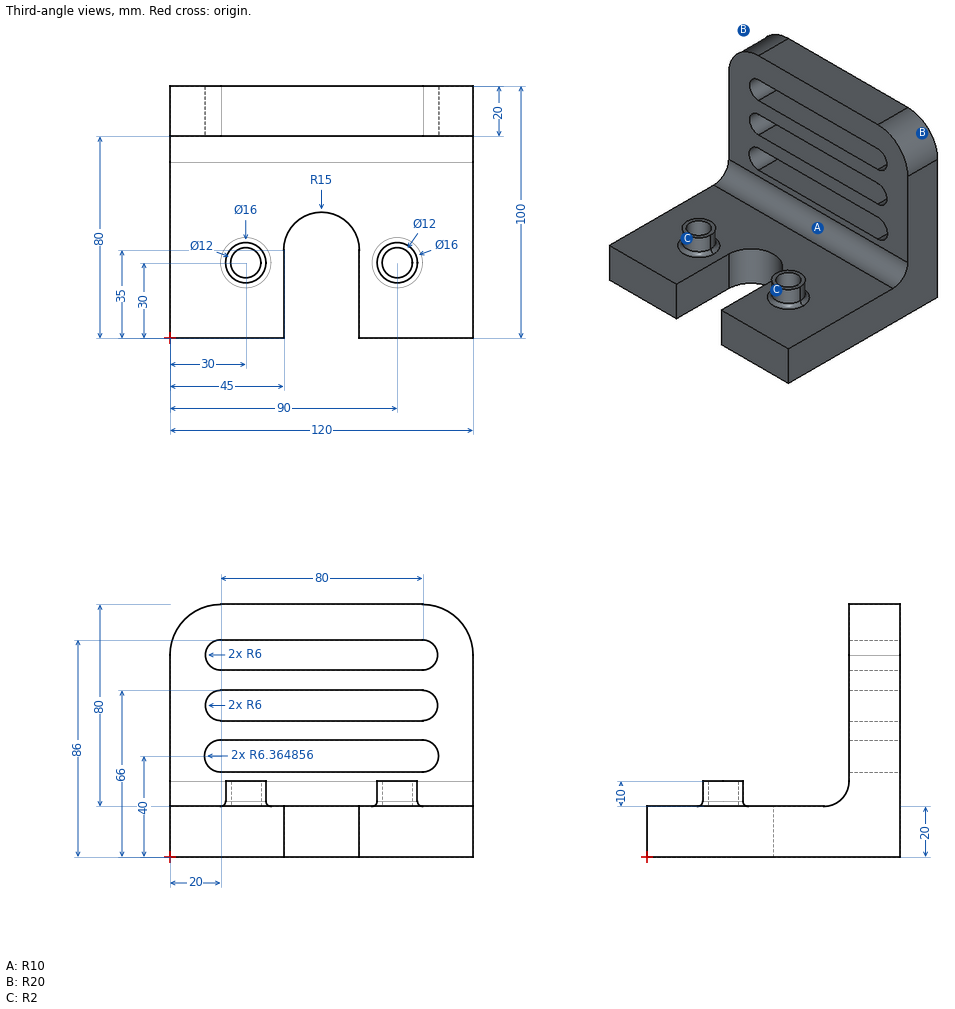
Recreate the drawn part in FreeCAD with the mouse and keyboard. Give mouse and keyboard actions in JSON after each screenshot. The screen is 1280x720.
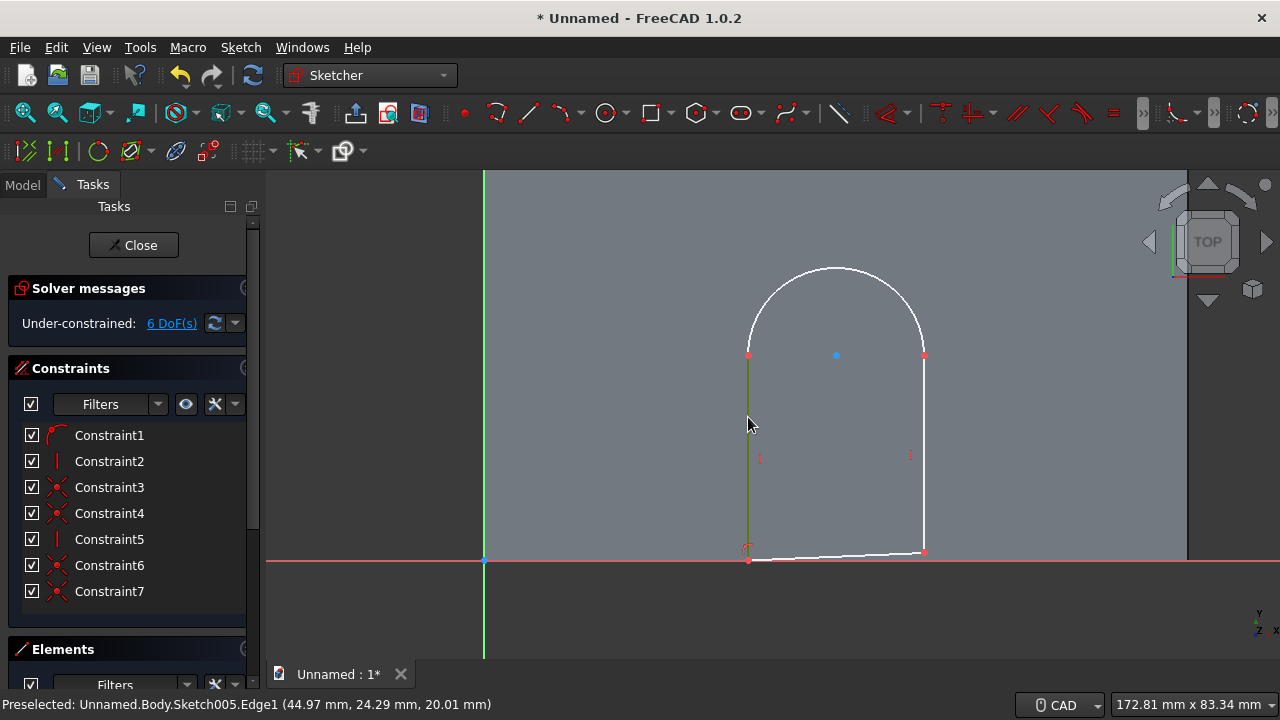
{"action": "left_click", "coordinate": [888, 285]}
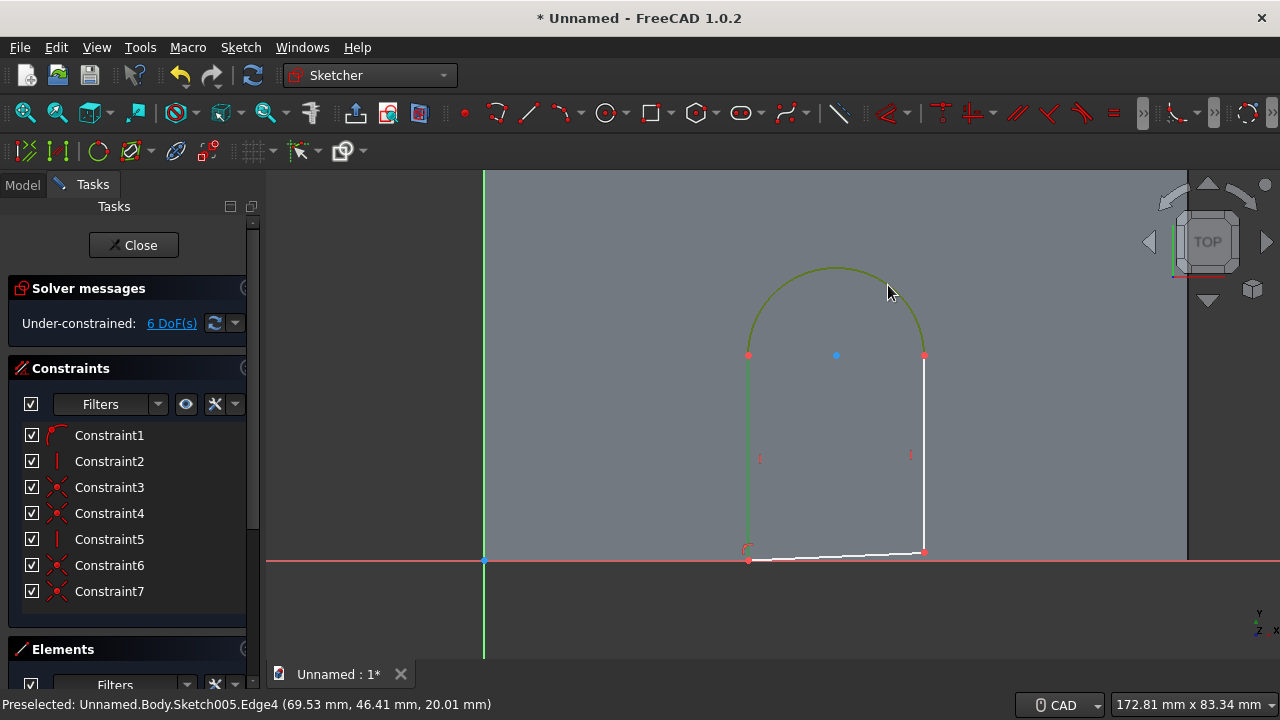
{"action": "left_click", "coordinate": [1082, 114]}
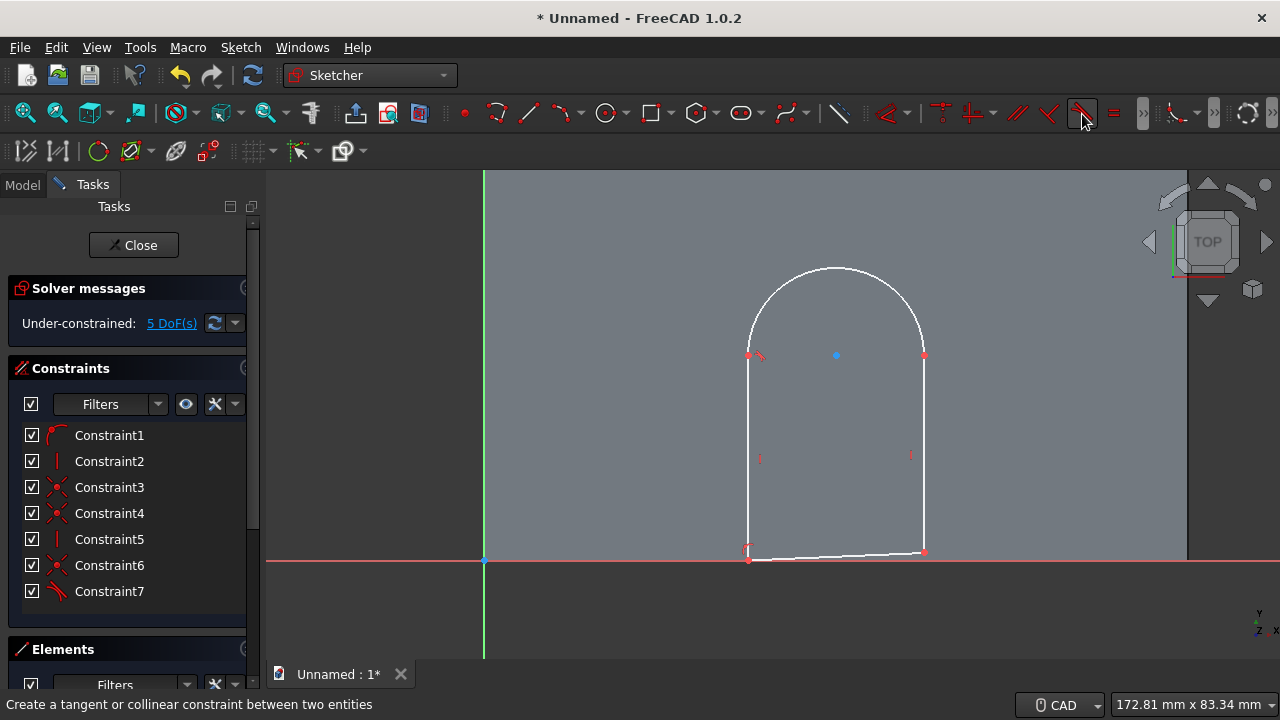
{"action": "left_click", "coordinate": [924, 494]}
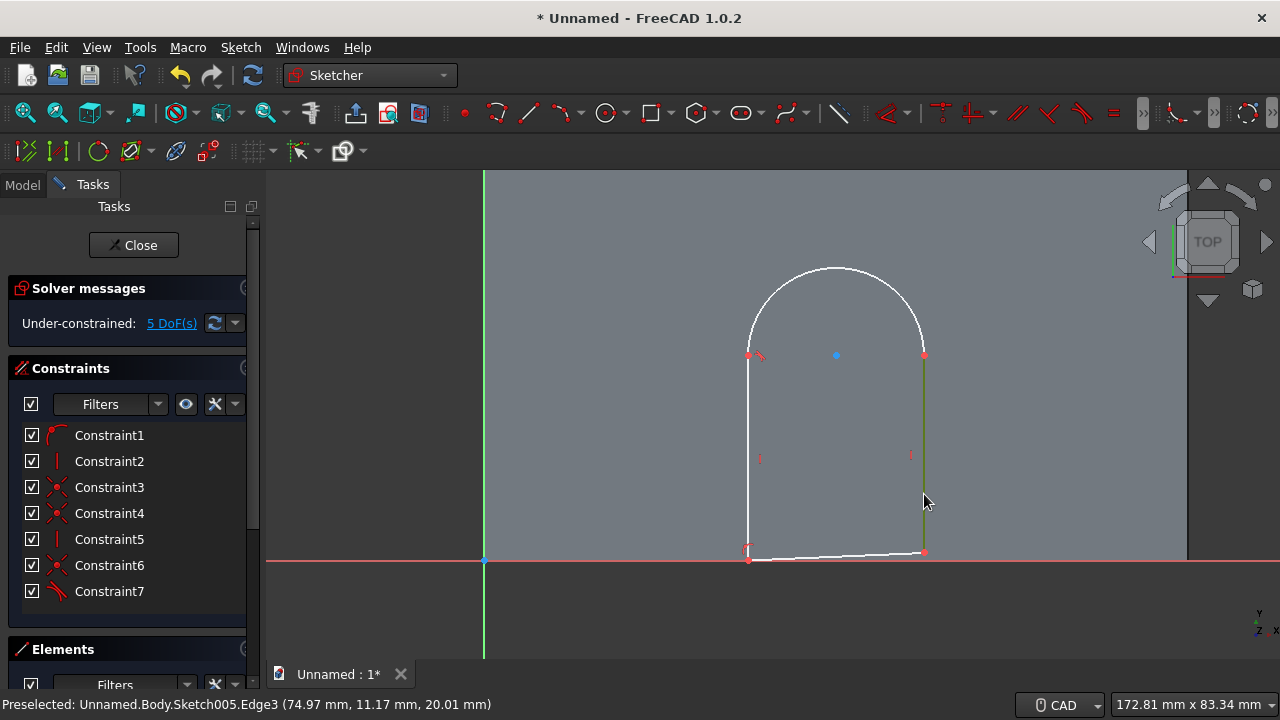
{"action": "left_click", "coordinate": [888, 285]}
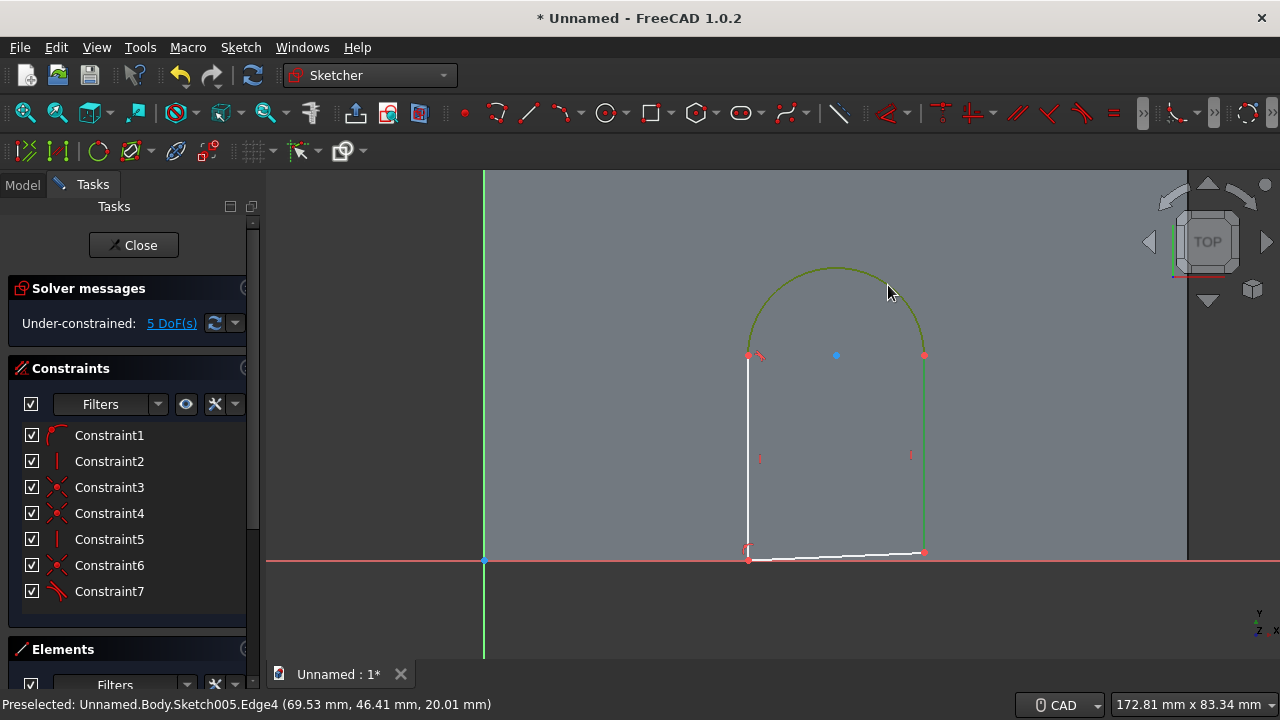
{"action": "key", "text": "t"}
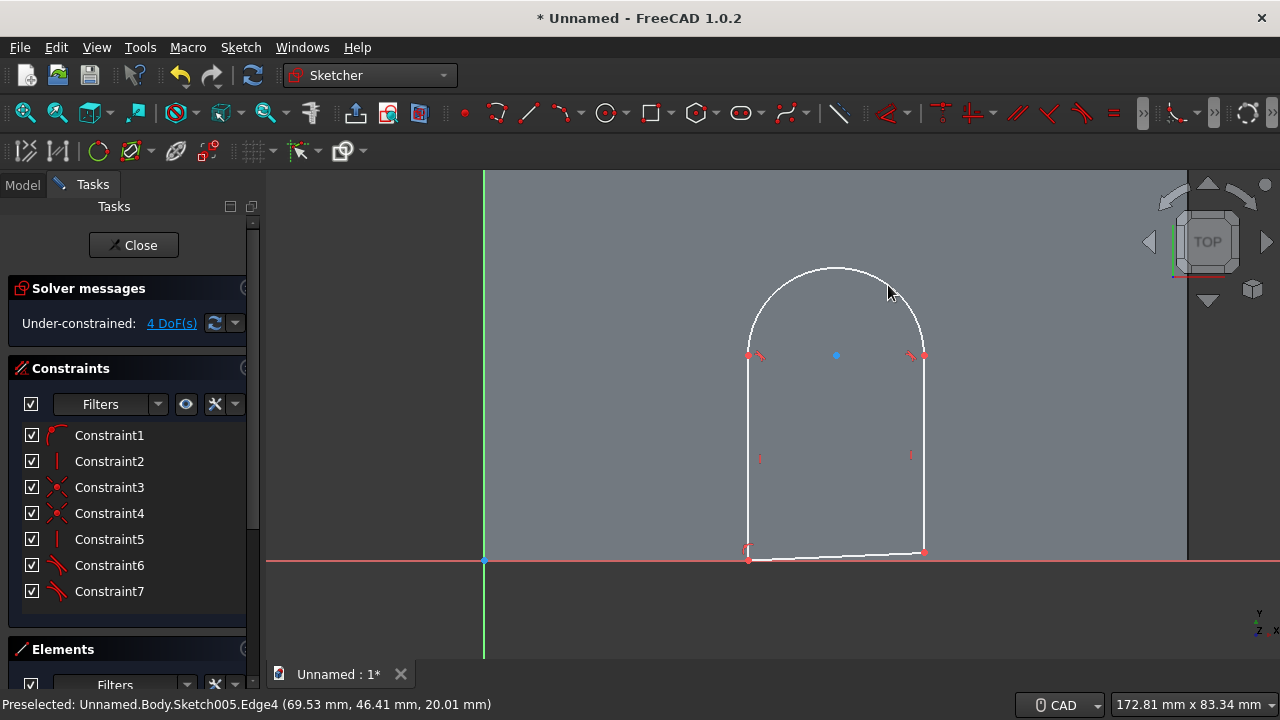
{"action": "left_click", "coordinate": [801, 558]}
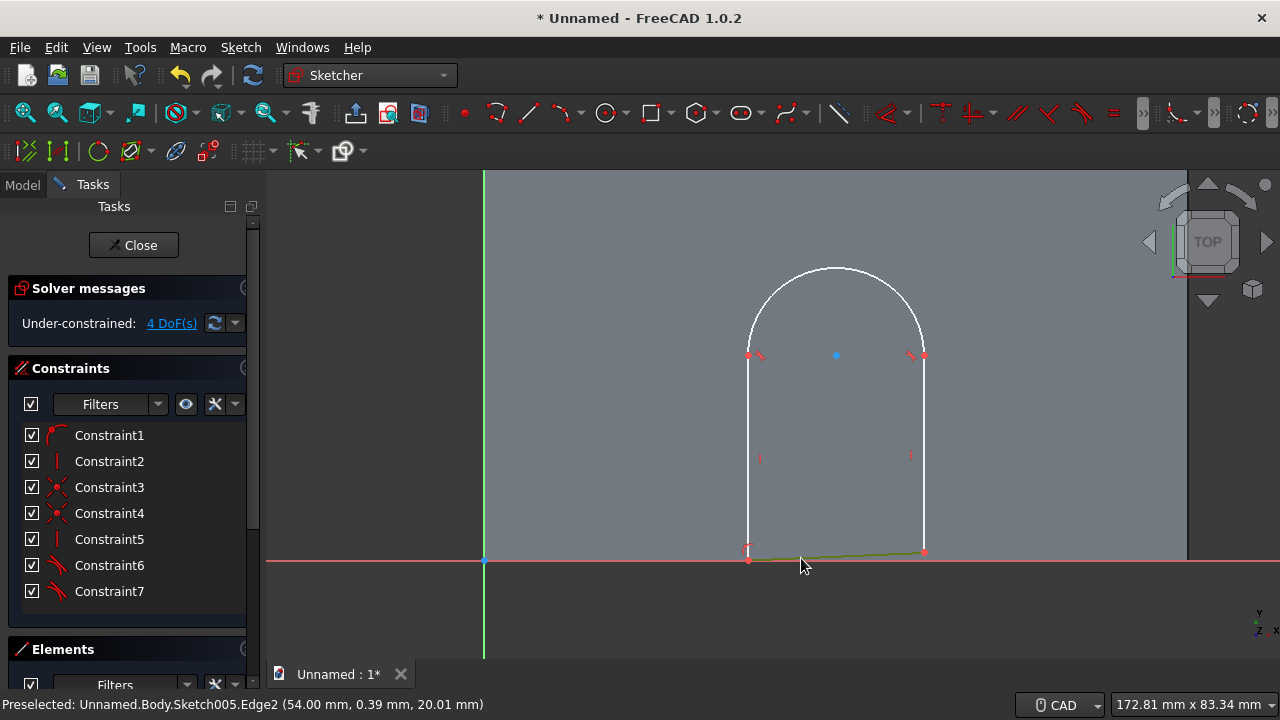
{"action": "key", "text": "h"}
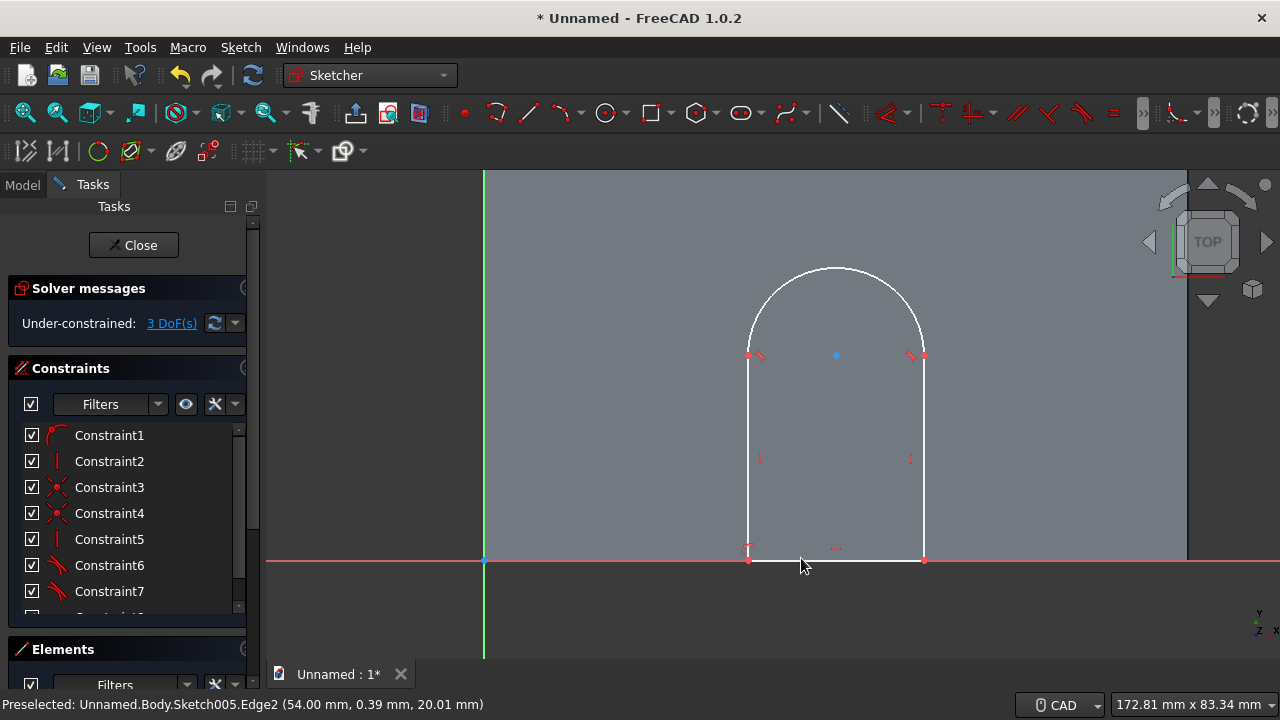
{"action": "key", "text": "d"}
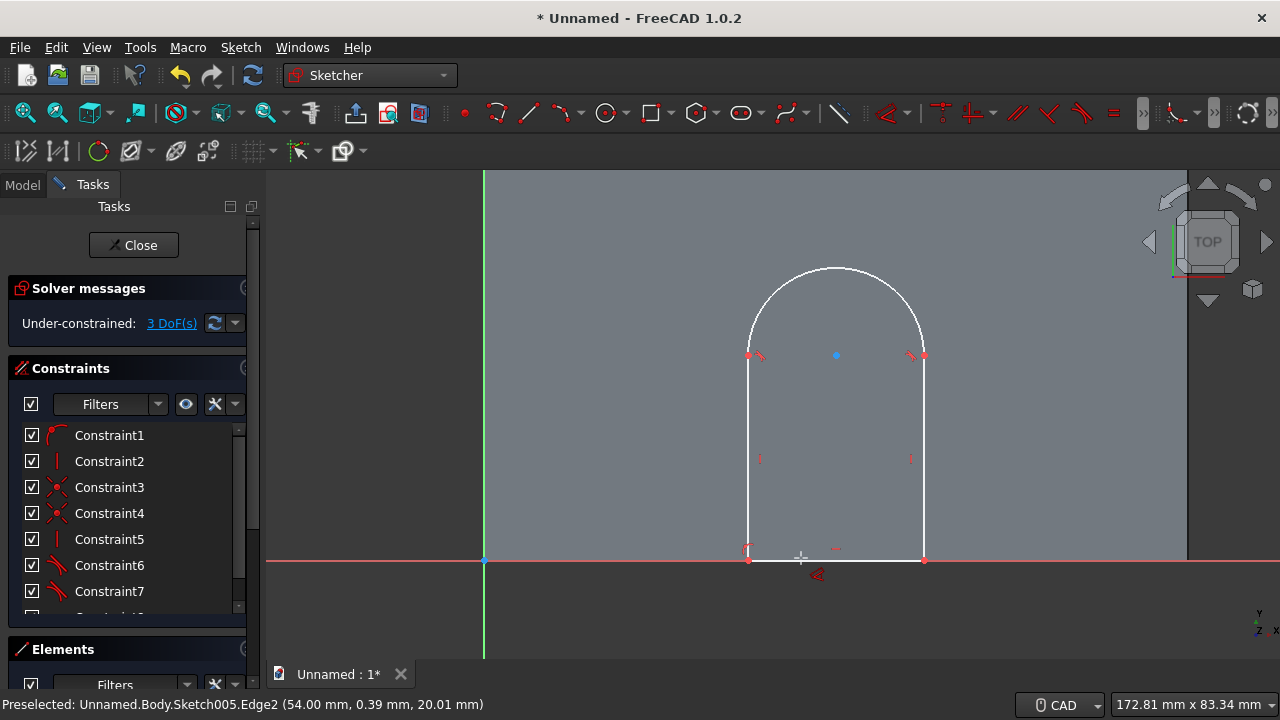
{"action": "left_click", "coordinate": [888, 285]}
{"action": "left_click", "coordinate": [907, 259]}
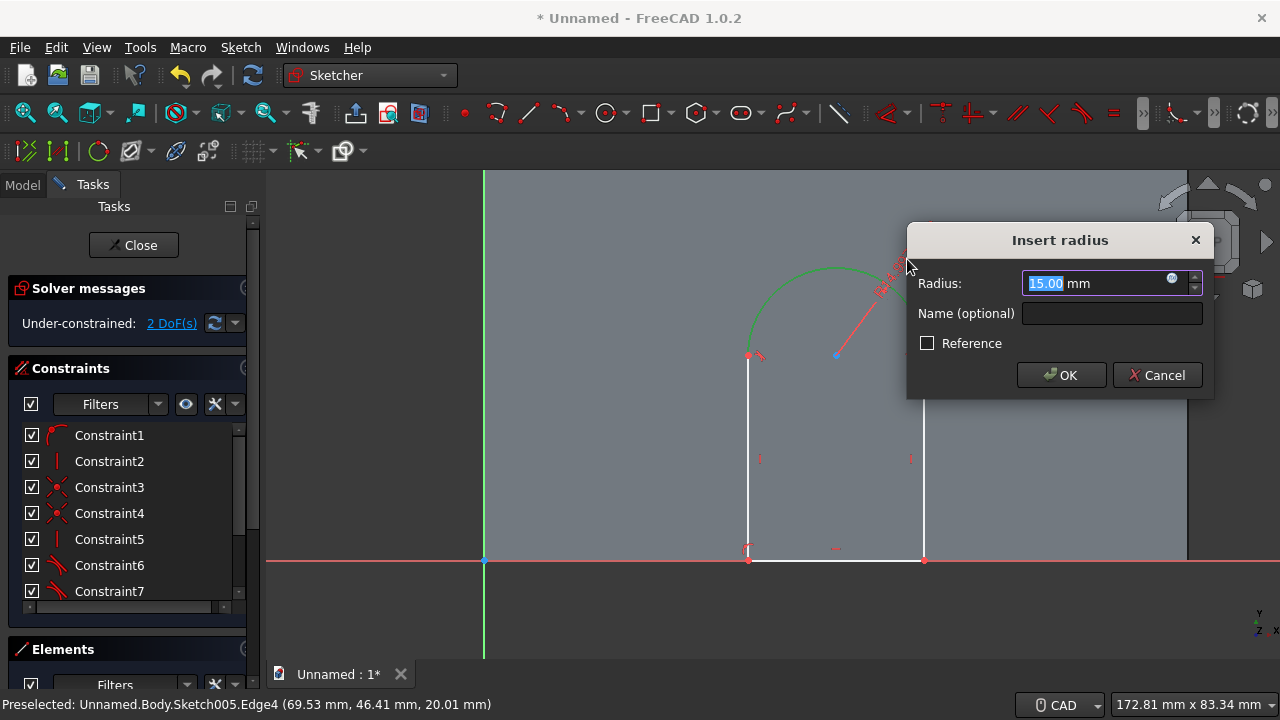
{"action": "type", "text": "15"}
{"action": "key", "text": "Return"}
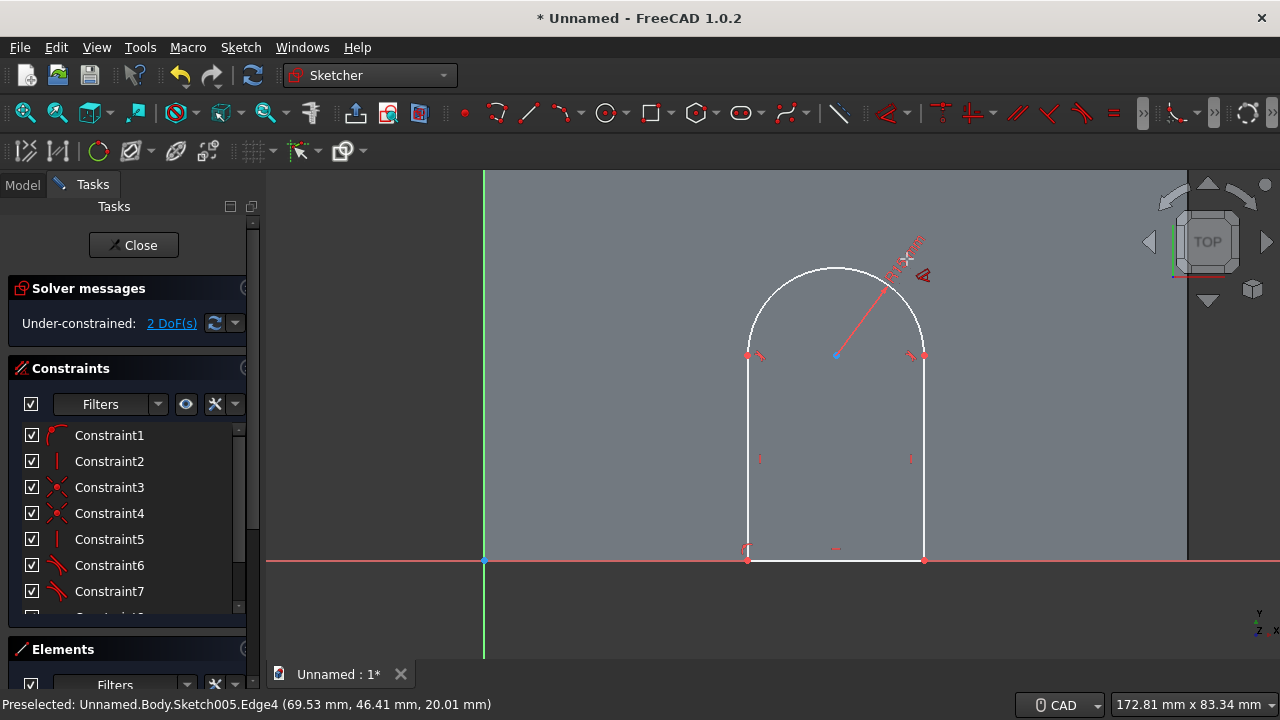
{"action": "left_click", "coordinate": [748, 417]}
{"action": "left_click", "coordinate": [782, 458]}